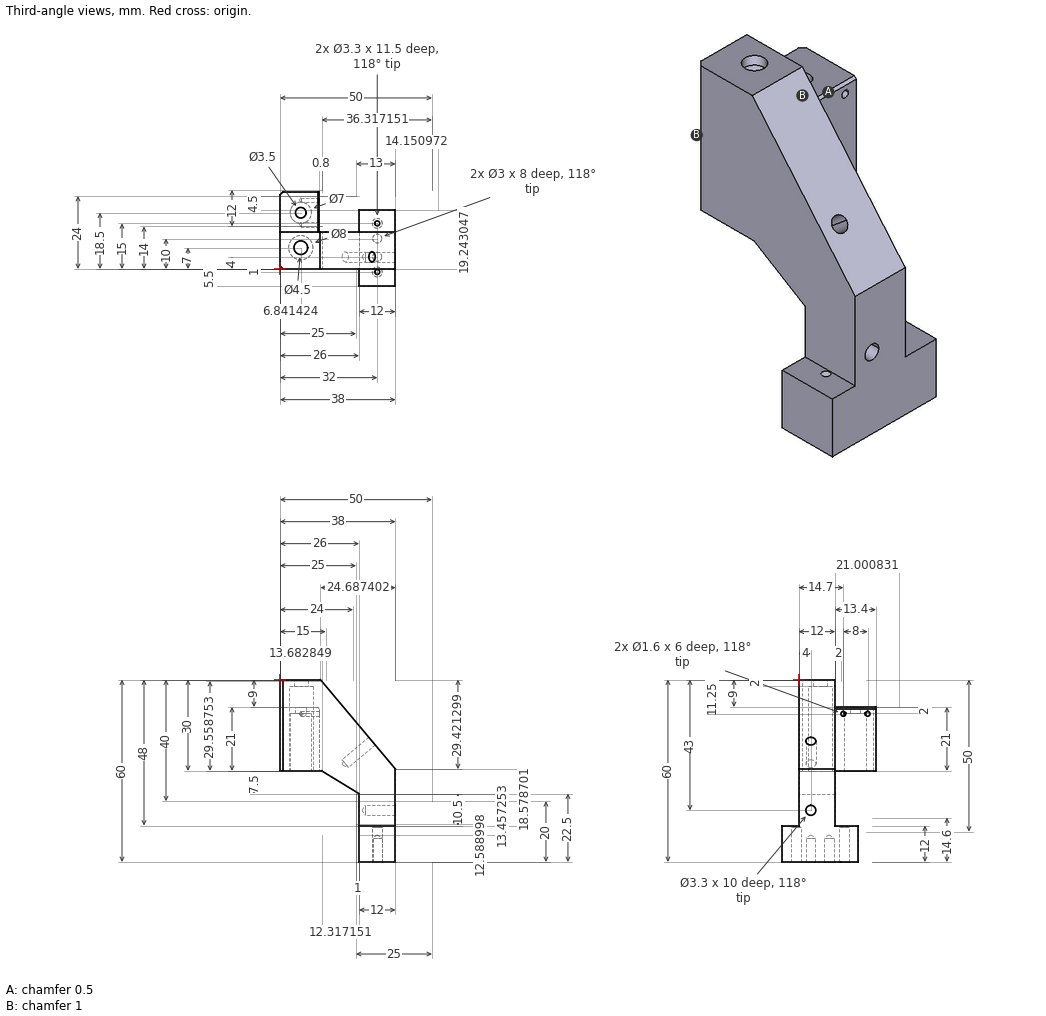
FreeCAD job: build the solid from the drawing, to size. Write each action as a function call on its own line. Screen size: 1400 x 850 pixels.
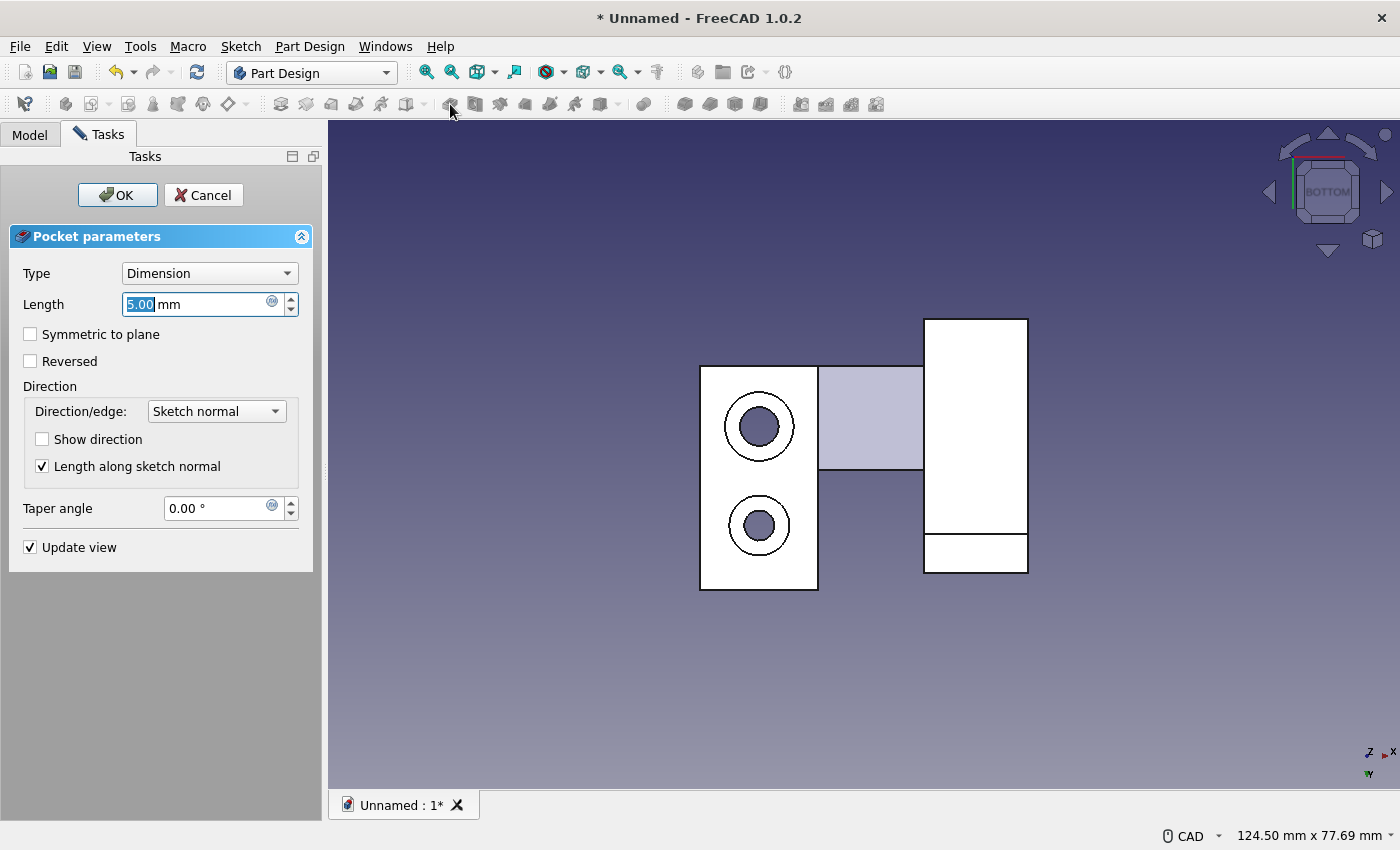
text(14.6)
key(Tab)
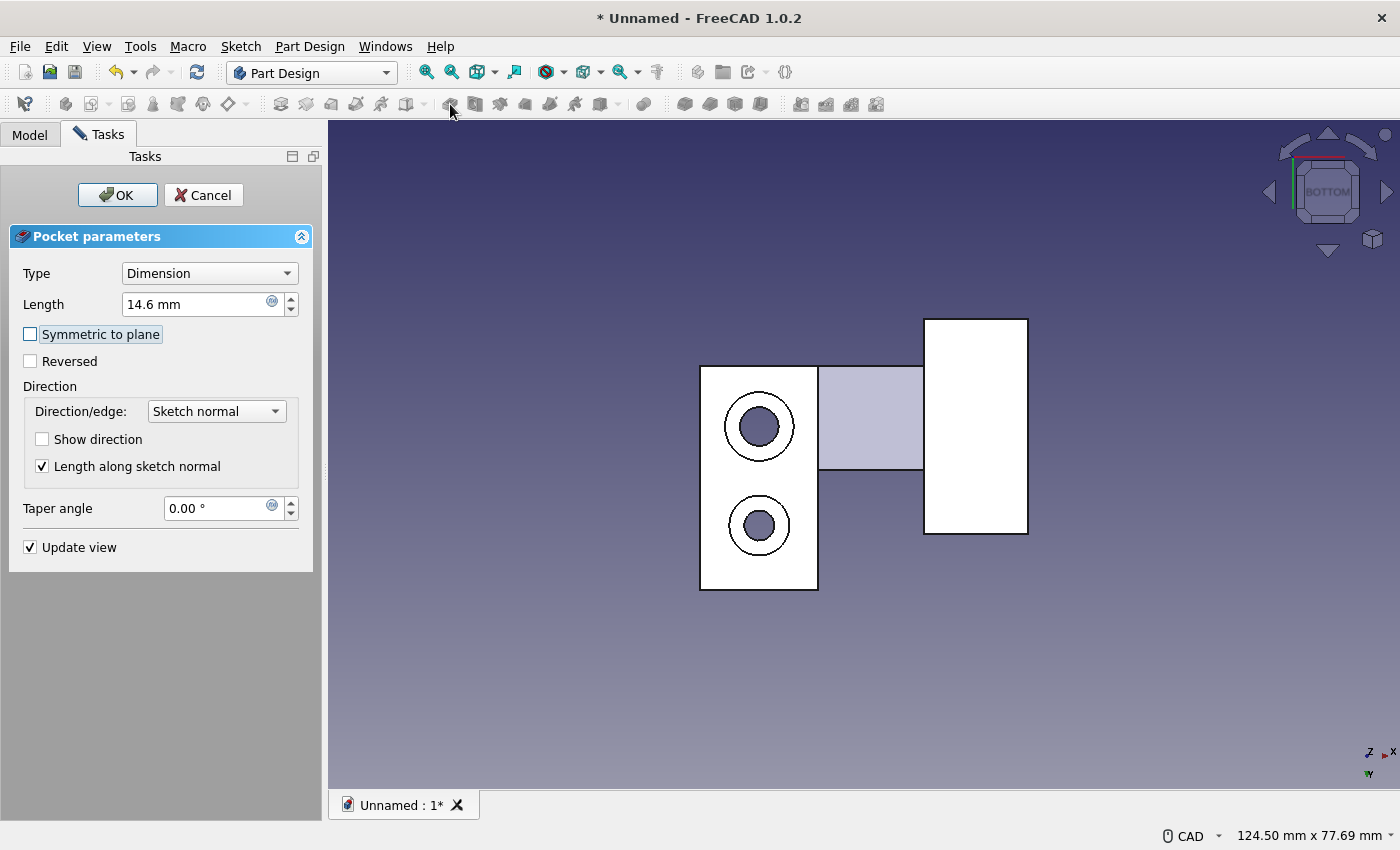
click(118, 195)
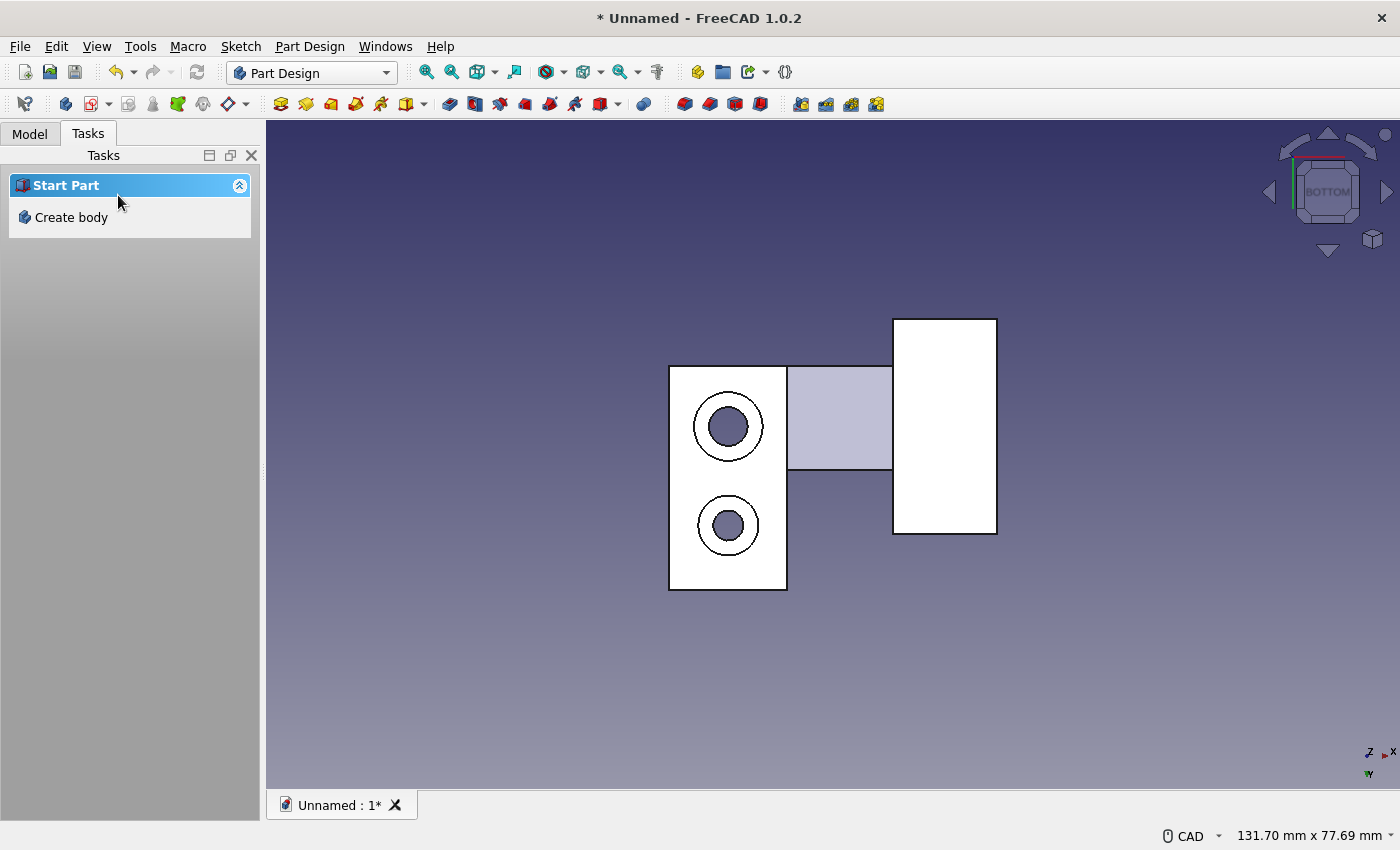
click(427, 72)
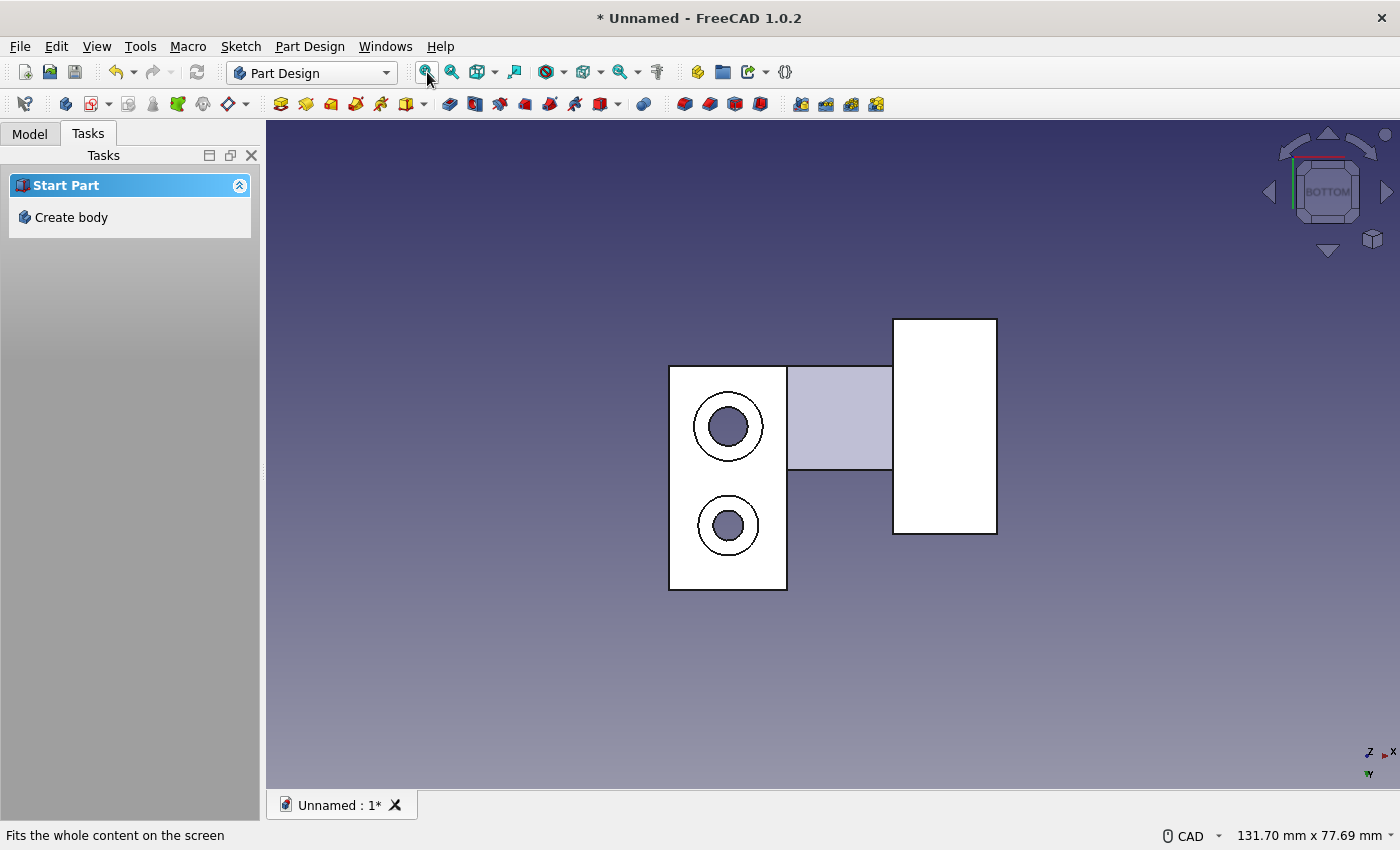
key(4)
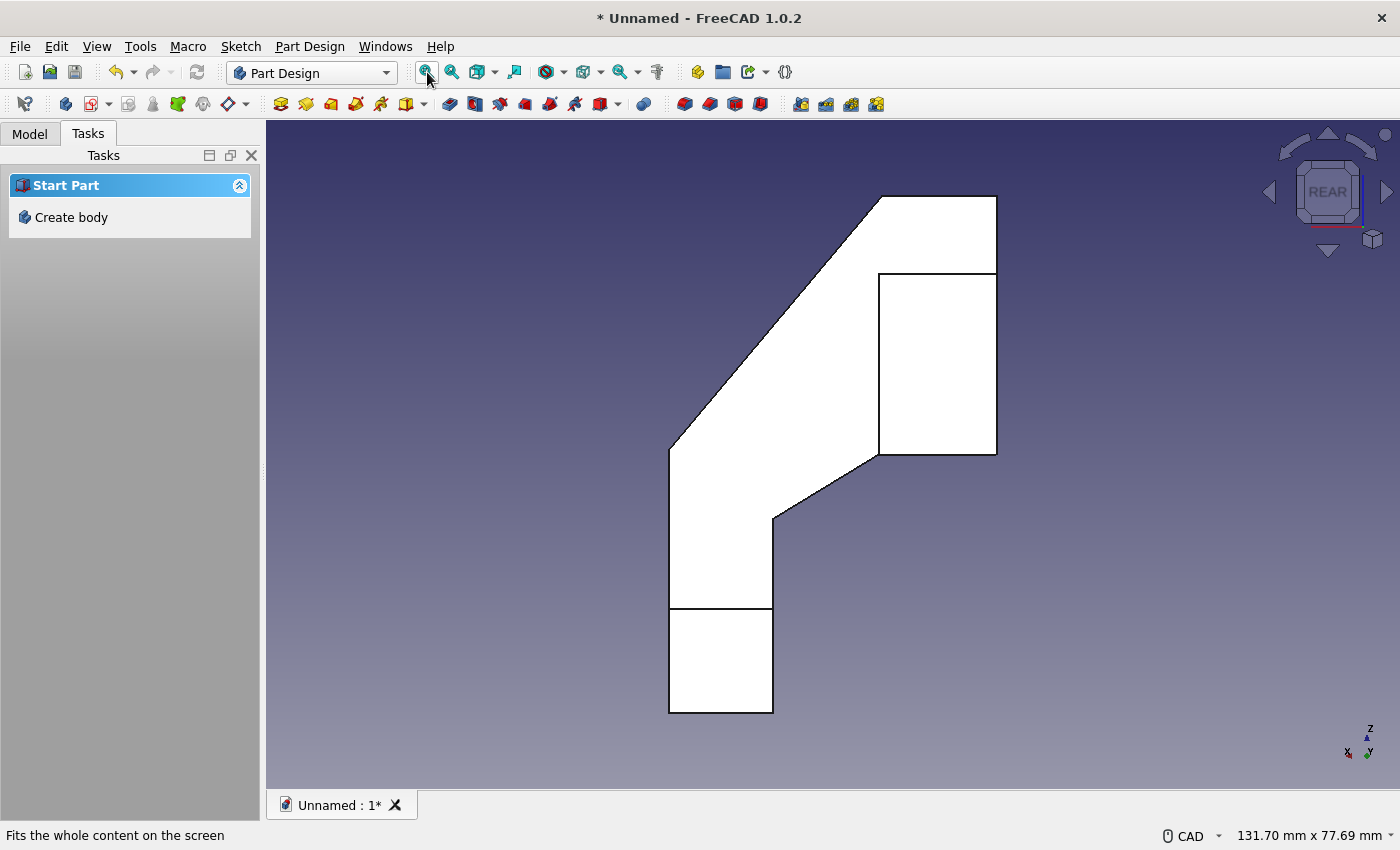
click(938, 337)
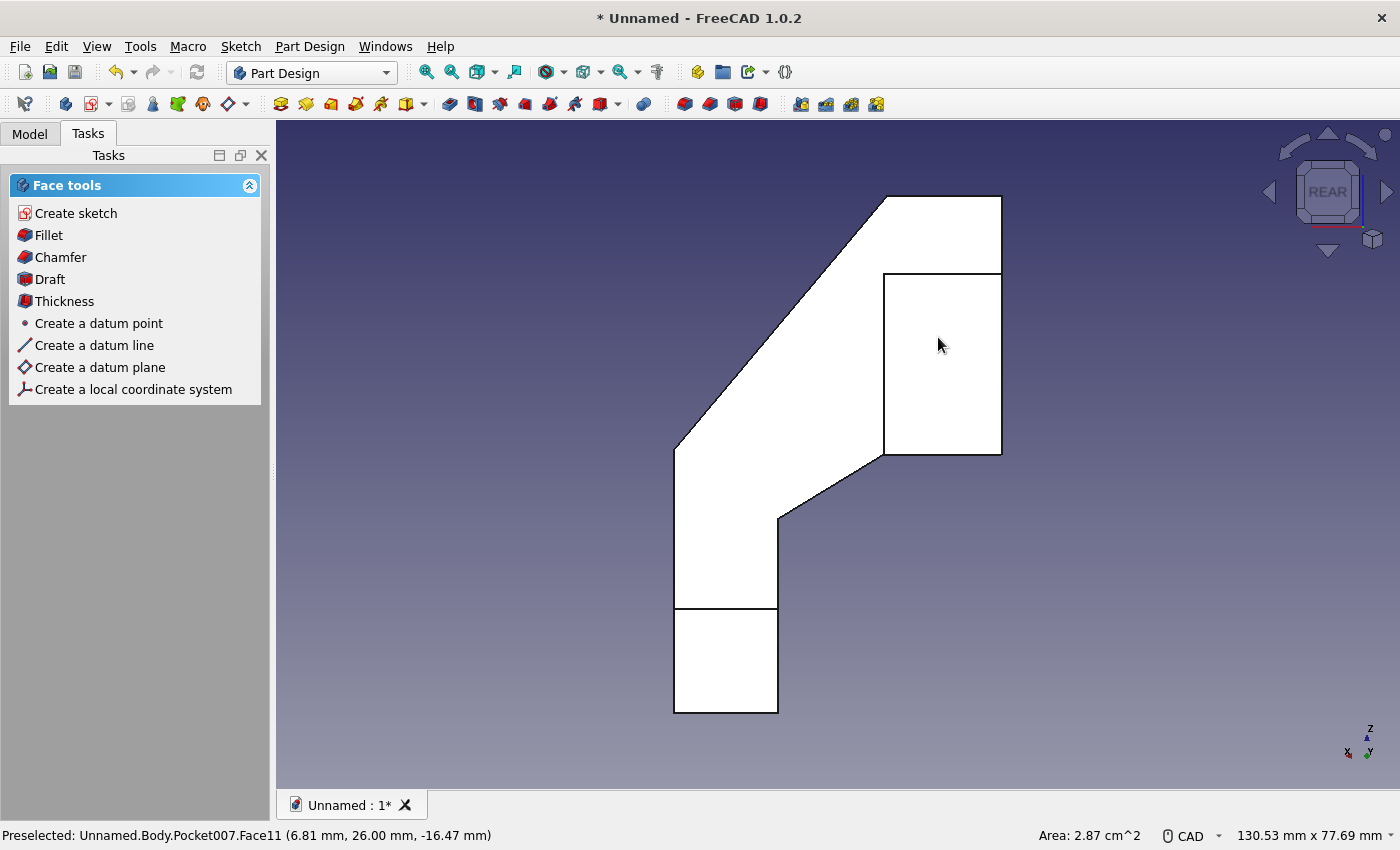
click(90, 104)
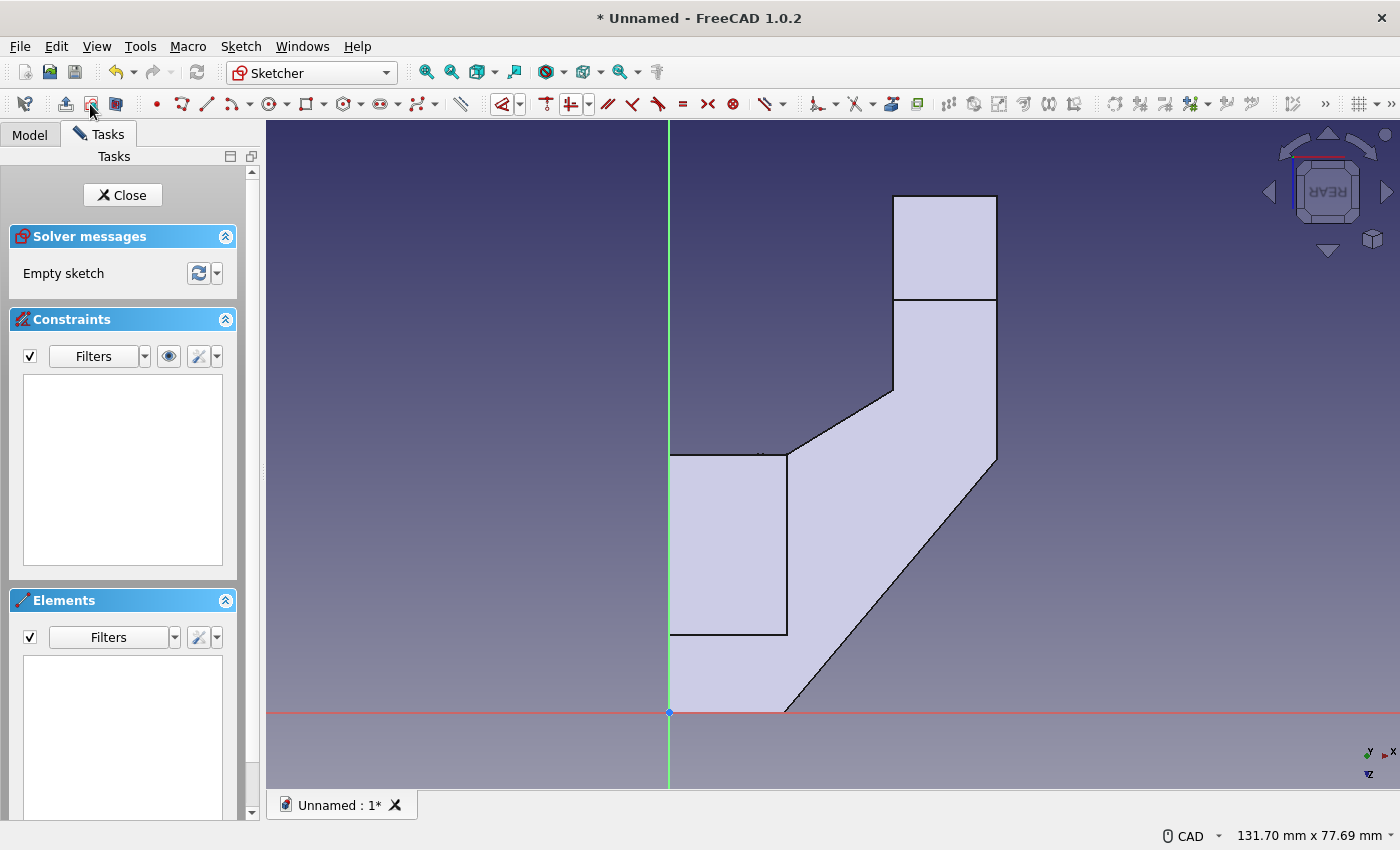
scroll(684, 741, up, 3)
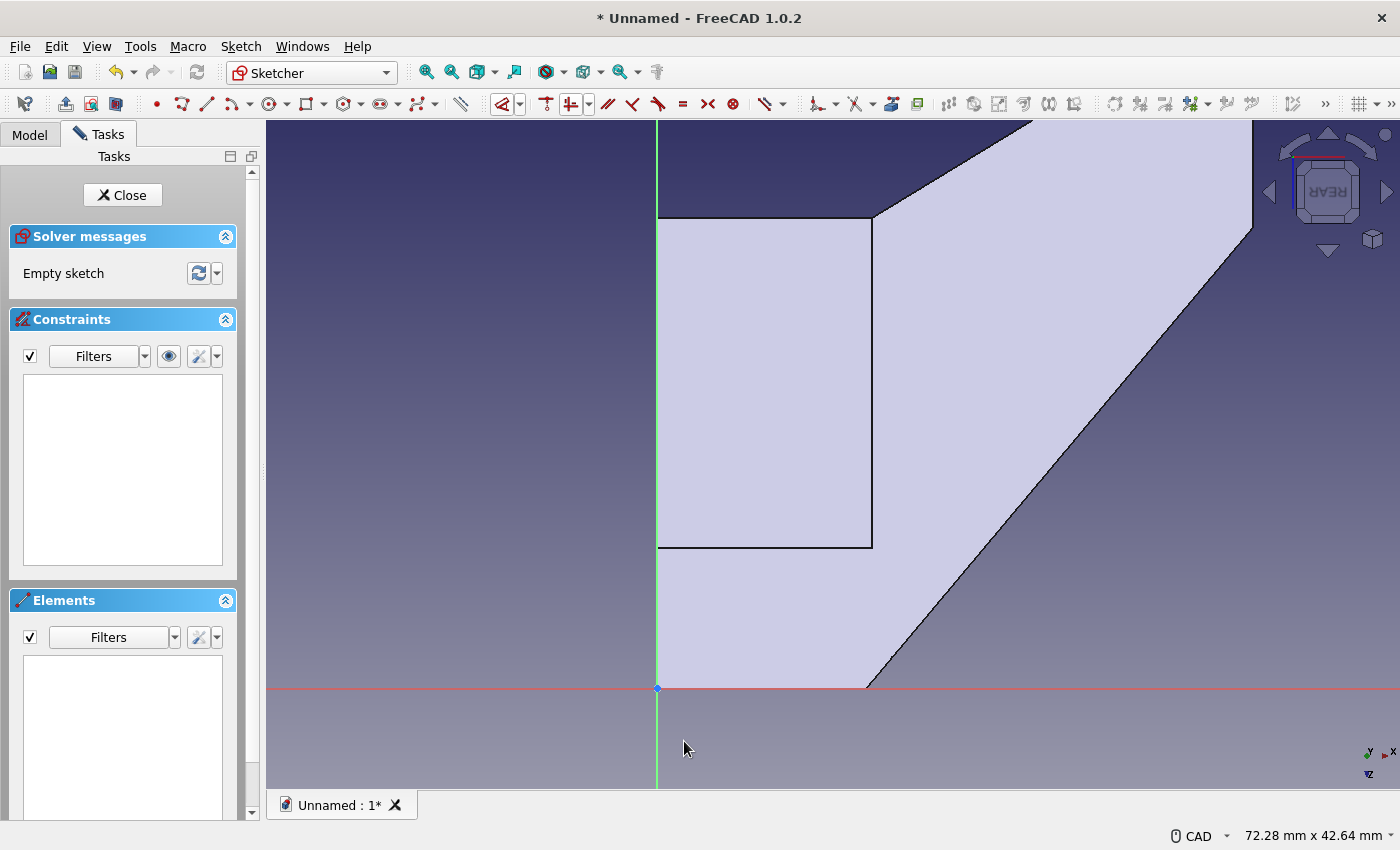
click(306, 104)